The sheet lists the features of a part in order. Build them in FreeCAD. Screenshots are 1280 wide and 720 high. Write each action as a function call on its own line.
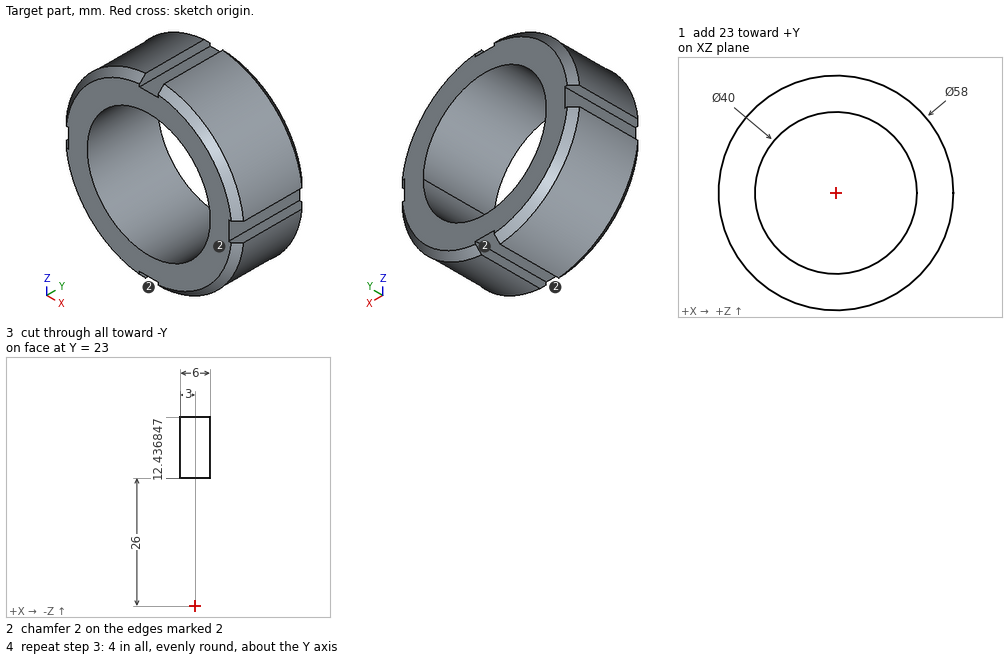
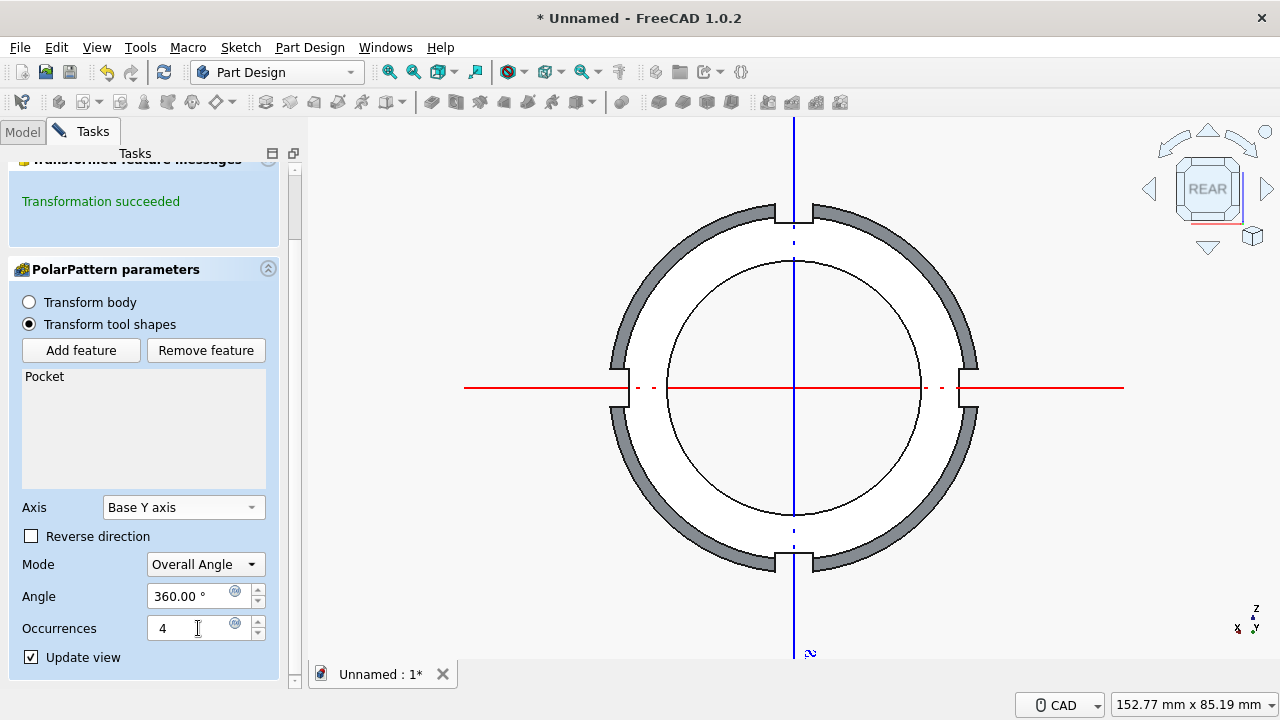
scroll(295, 426, up, 3)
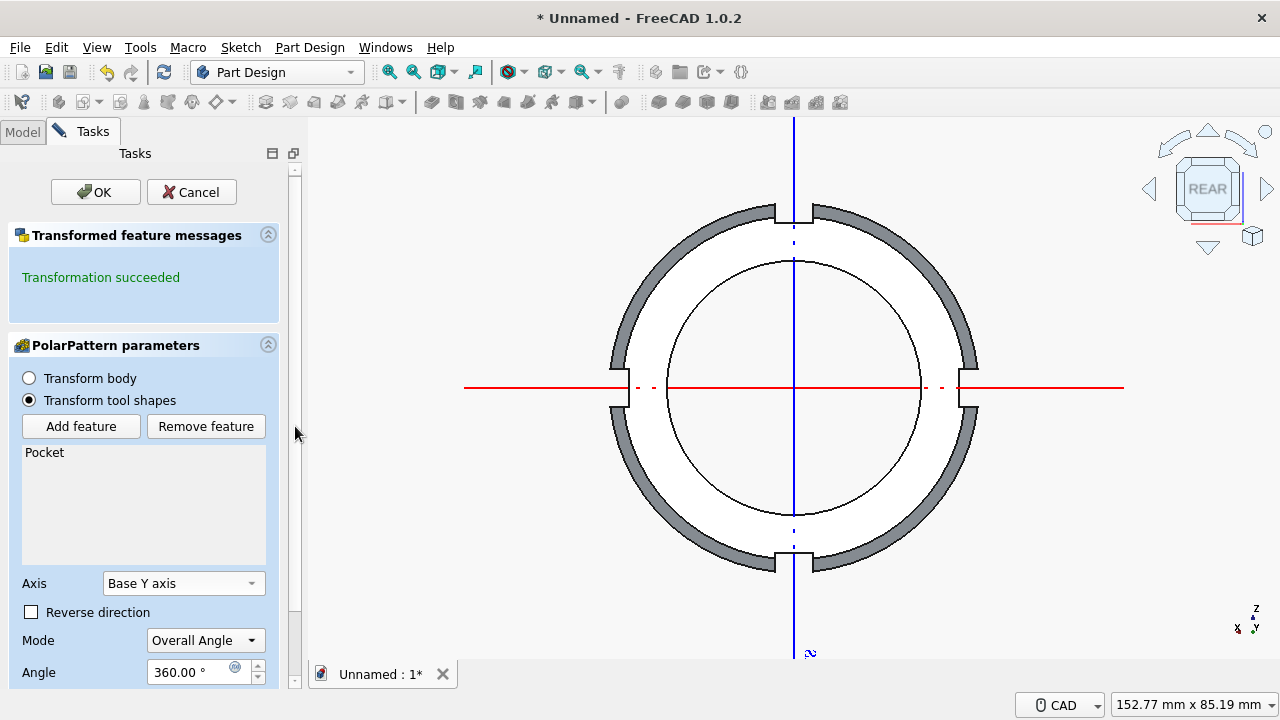
click(96, 192)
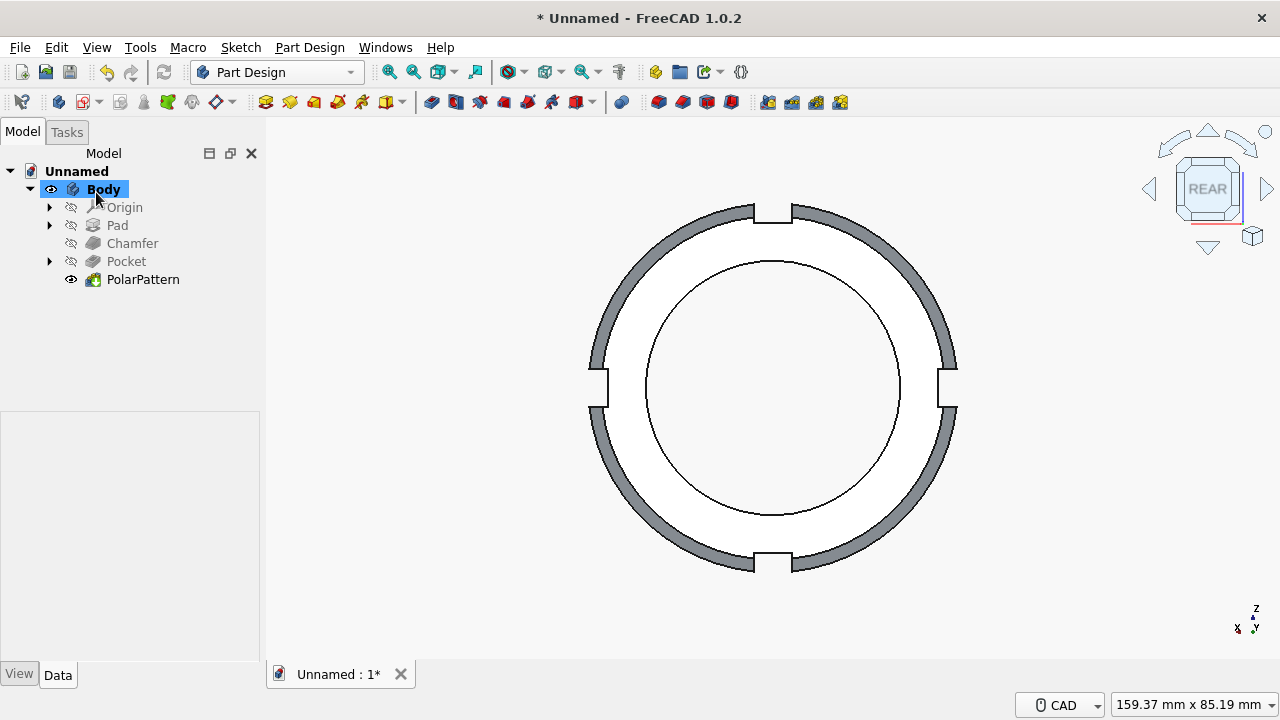
key(0)